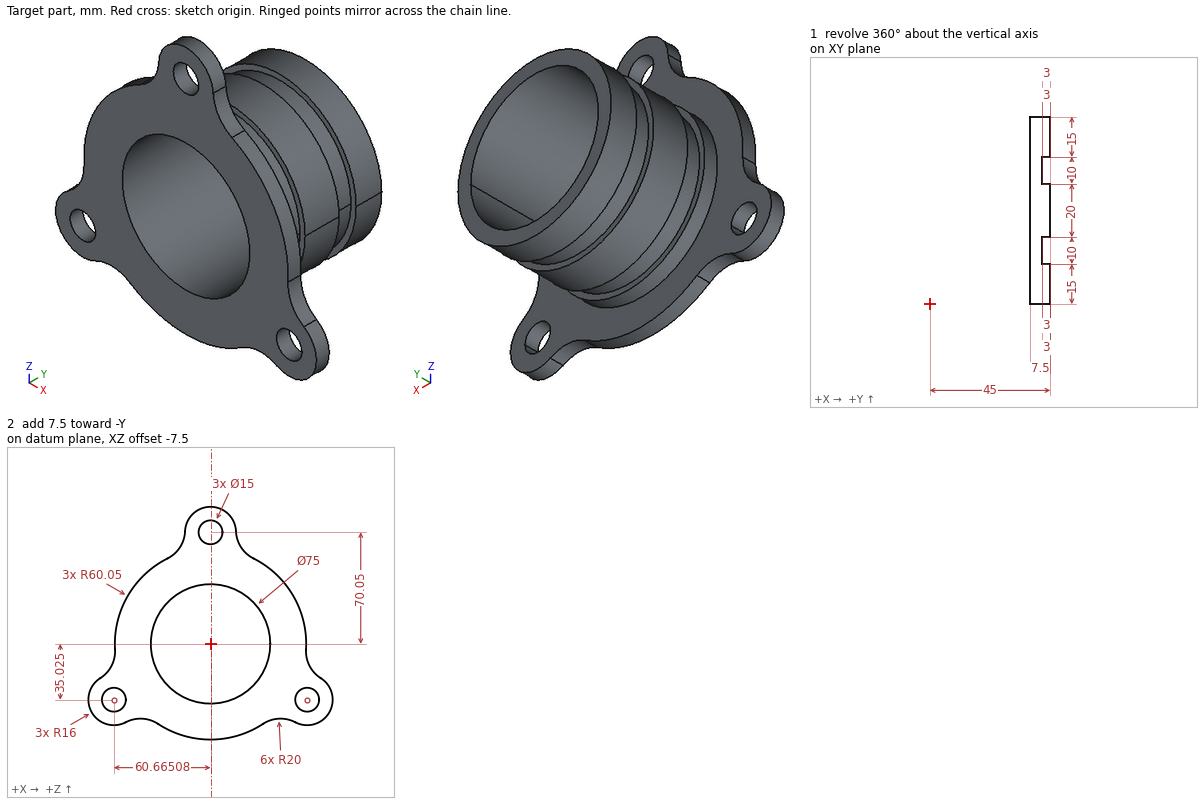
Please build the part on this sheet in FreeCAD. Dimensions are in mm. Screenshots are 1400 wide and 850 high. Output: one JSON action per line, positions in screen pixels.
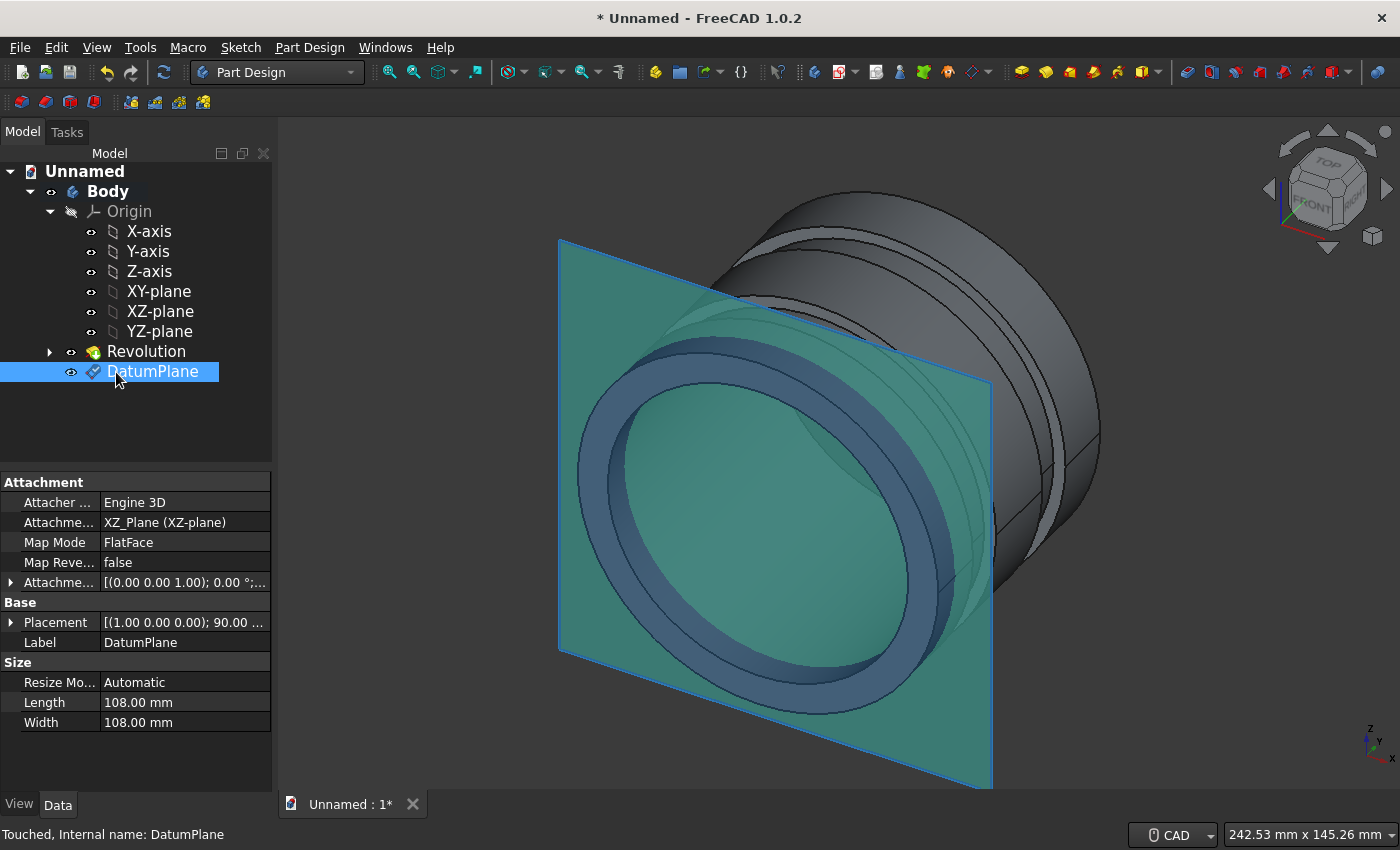
{"action": "left_click", "coordinate": [840, 72]}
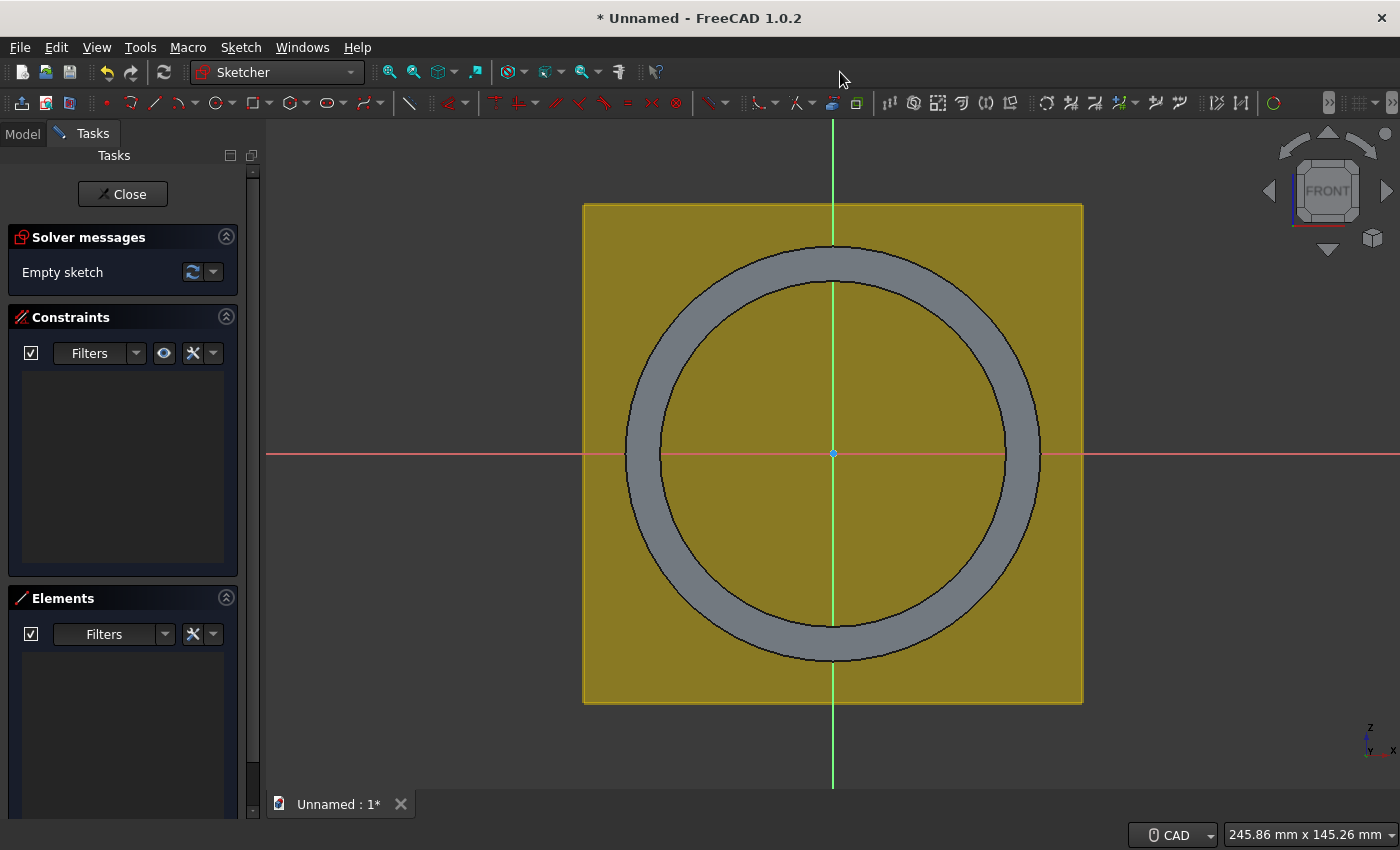
{"action": "left_click", "coordinate": [70, 104]}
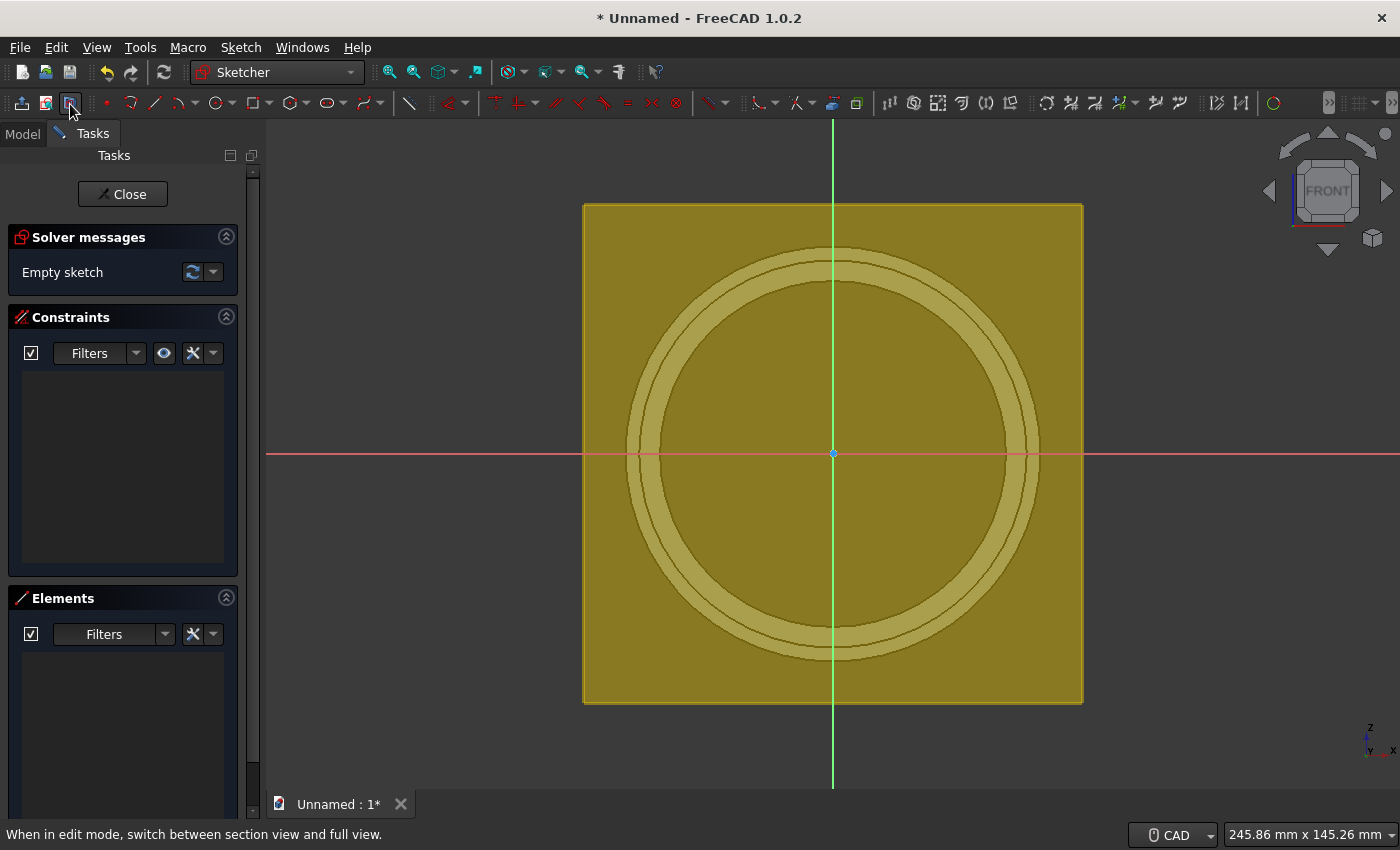
{"action": "scroll", "coordinate": [625, 576], "scroll_direction": "down", "scroll_amount": 2}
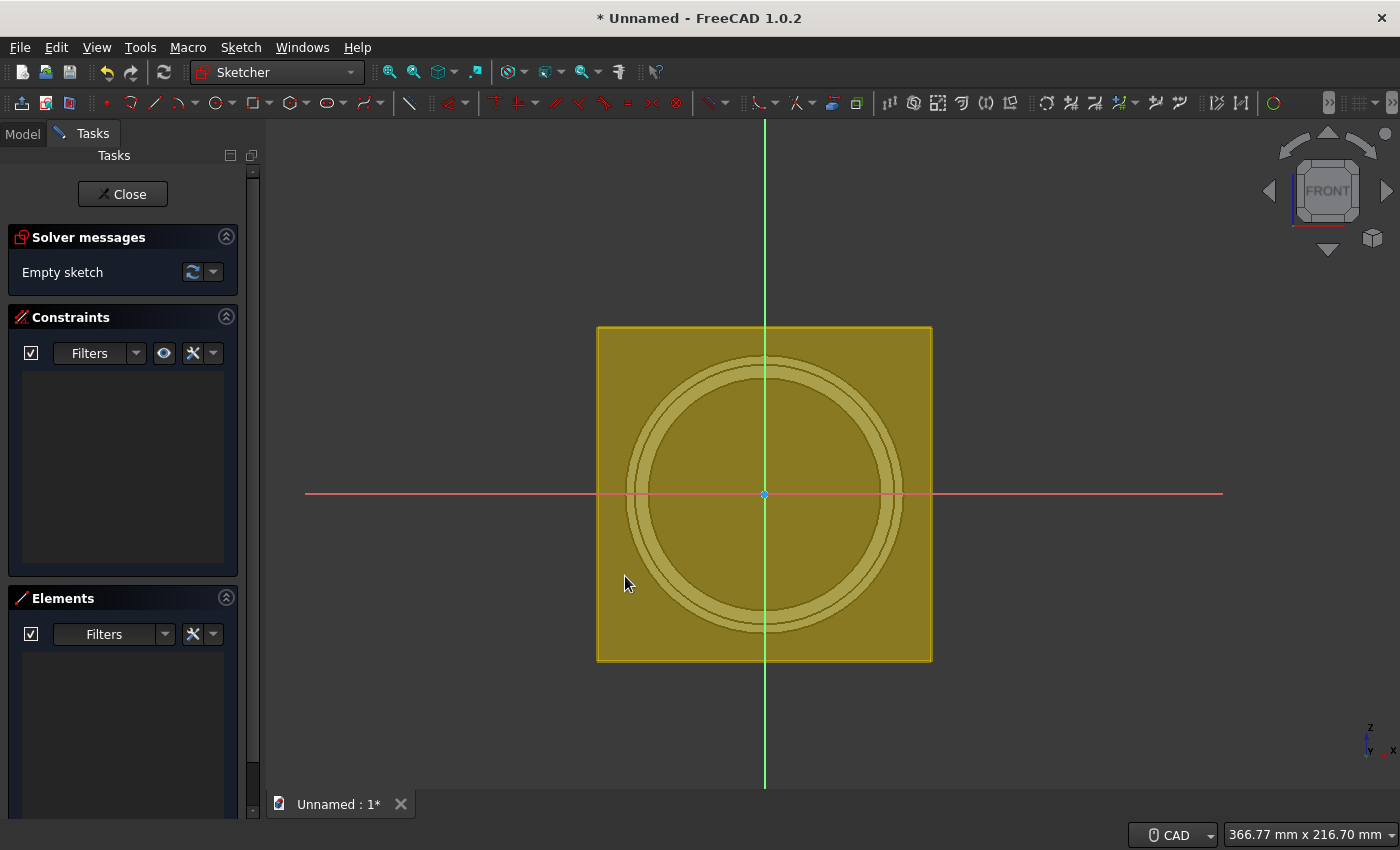
{"action": "key", "text": "g 3 a"}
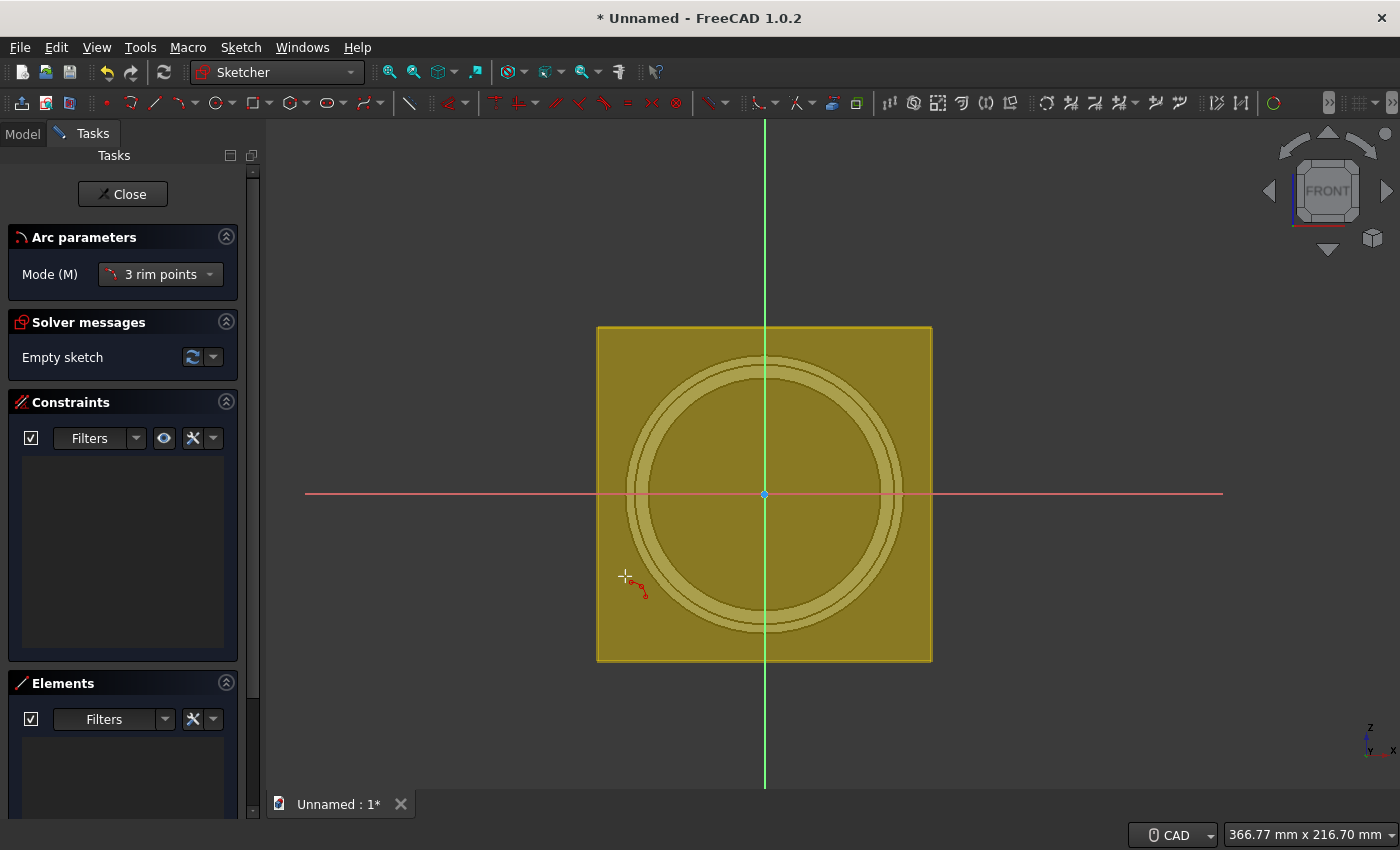
{"action": "scroll", "coordinate": [579, 505], "scroll_direction": "up", "scroll_amount": 2}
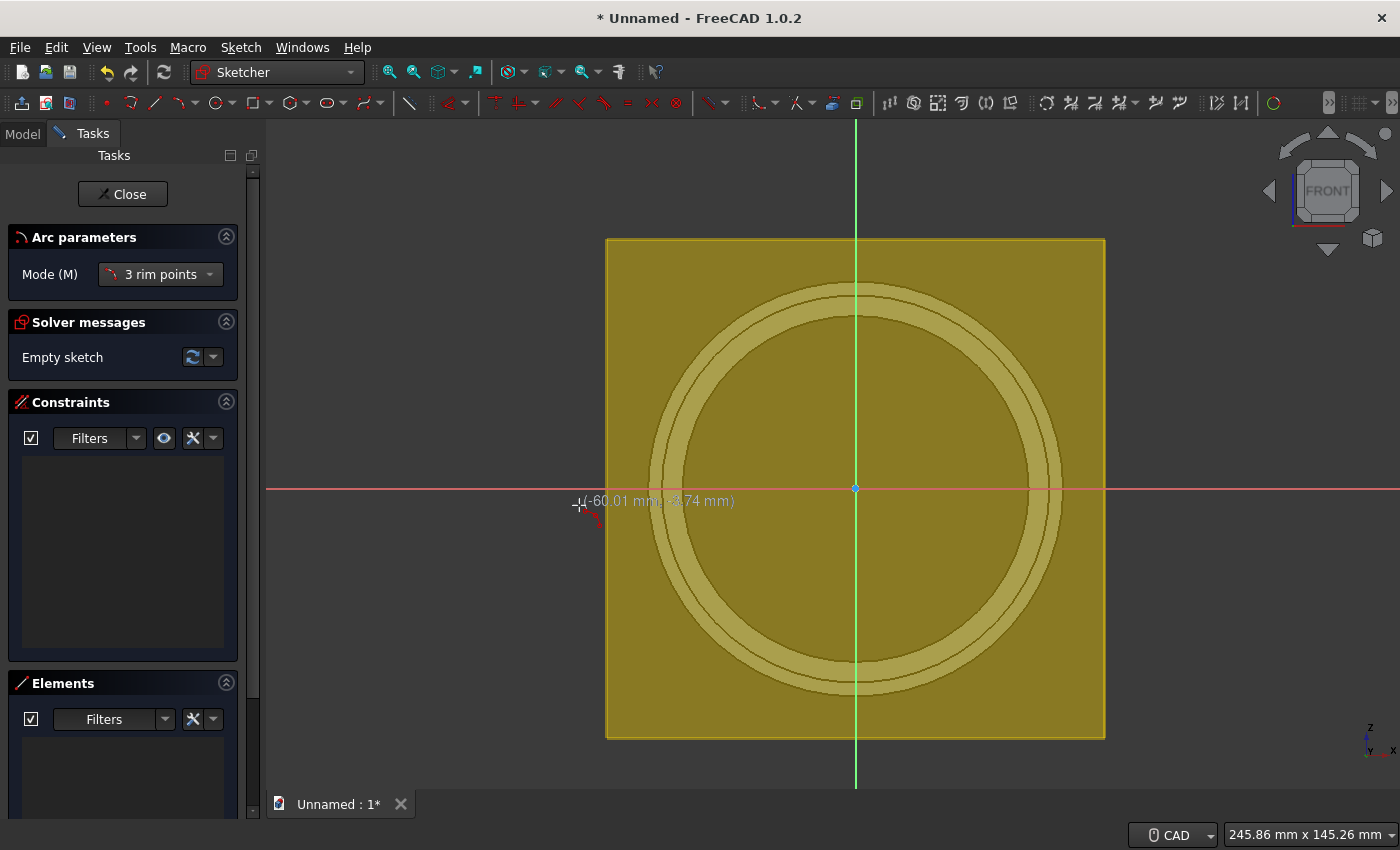
{"action": "left_click", "coordinate": [579, 505]}
{"action": "left_click", "coordinate": [536, 588]}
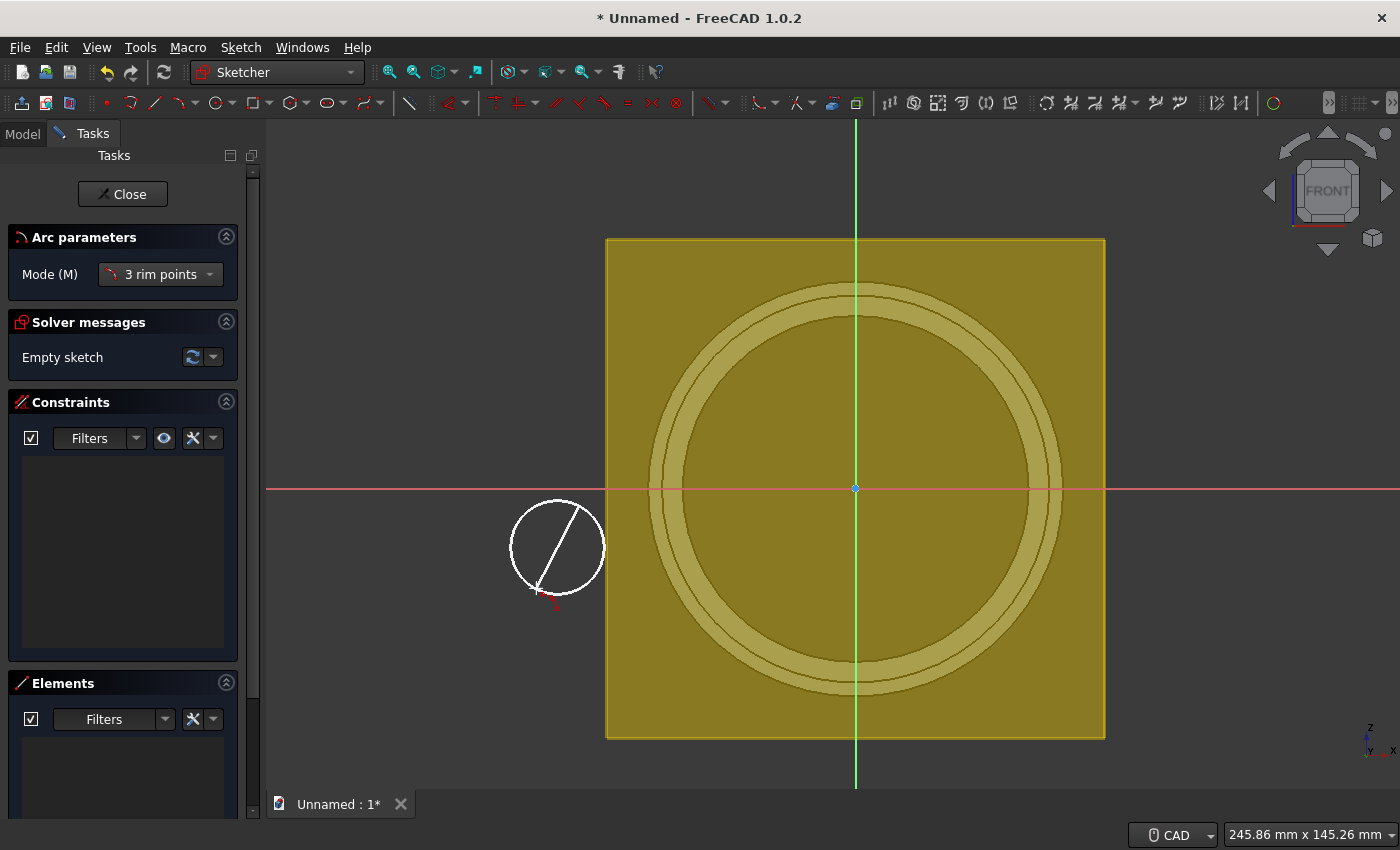
{"action": "scroll", "coordinate": [569, 552], "scroll_direction": "up", "scroll_amount": 2}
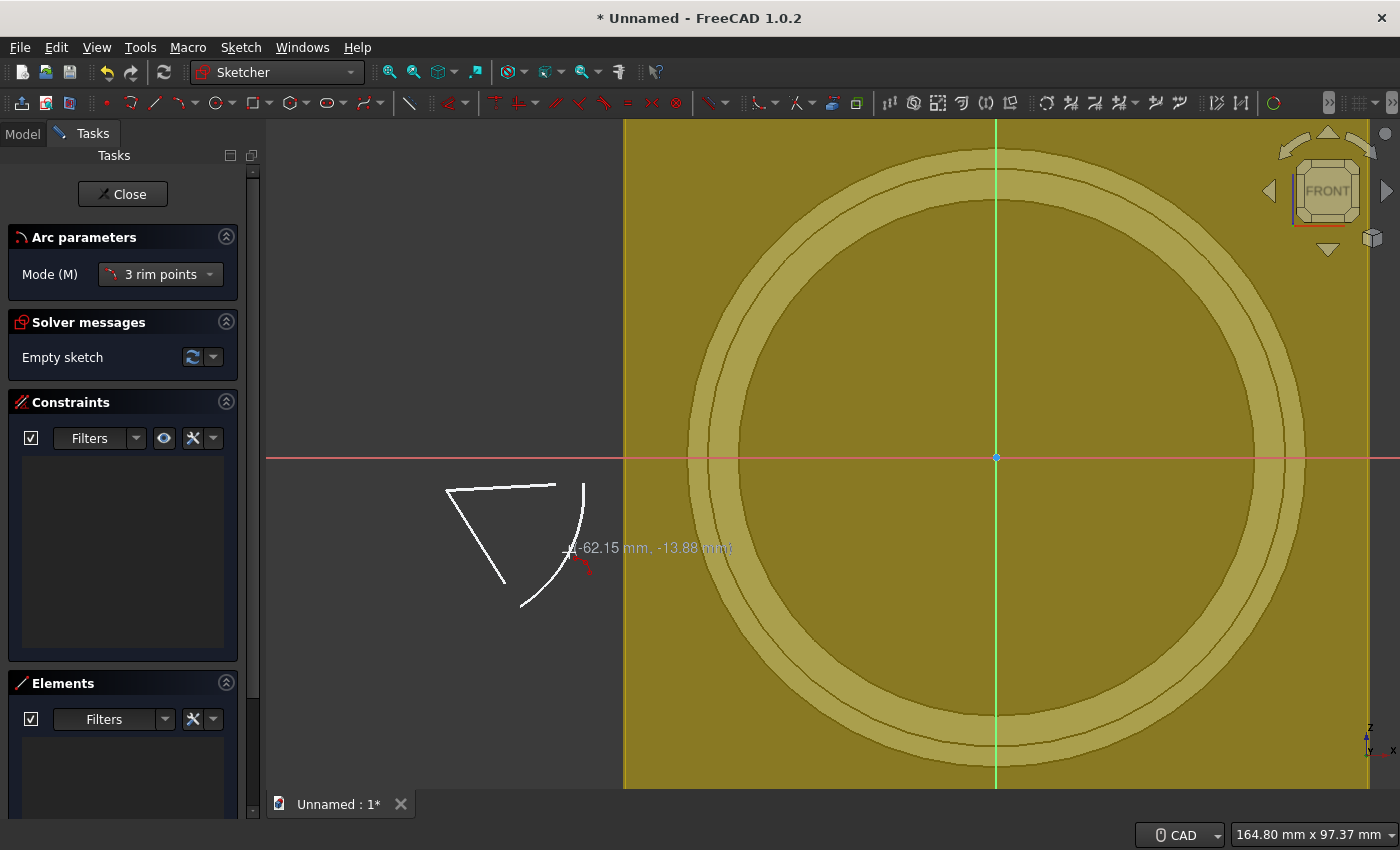
{"action": "left_click", "coordinate": [569, 552]}